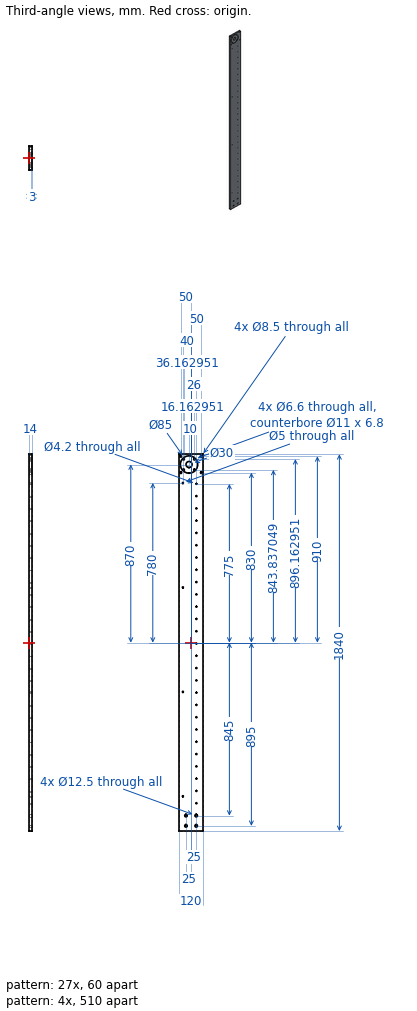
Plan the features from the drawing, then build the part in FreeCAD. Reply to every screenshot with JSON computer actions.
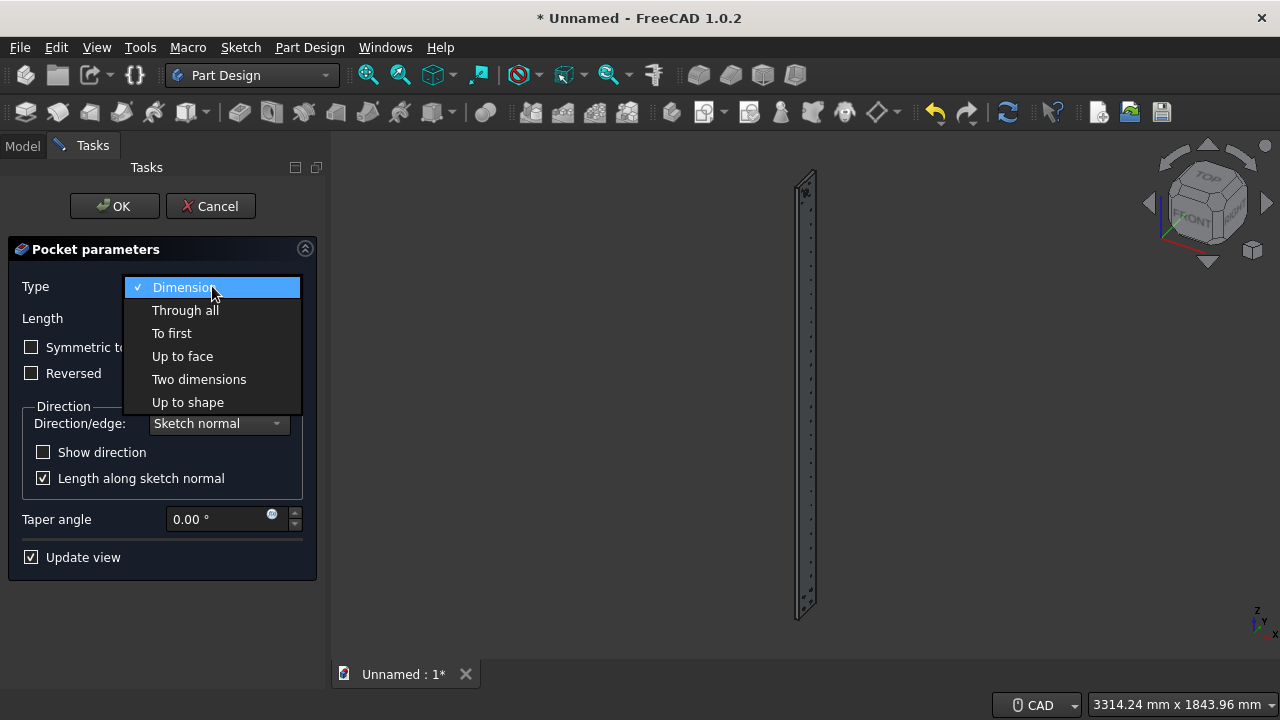
{"action": "left_click", "coordinate": [212, 310]}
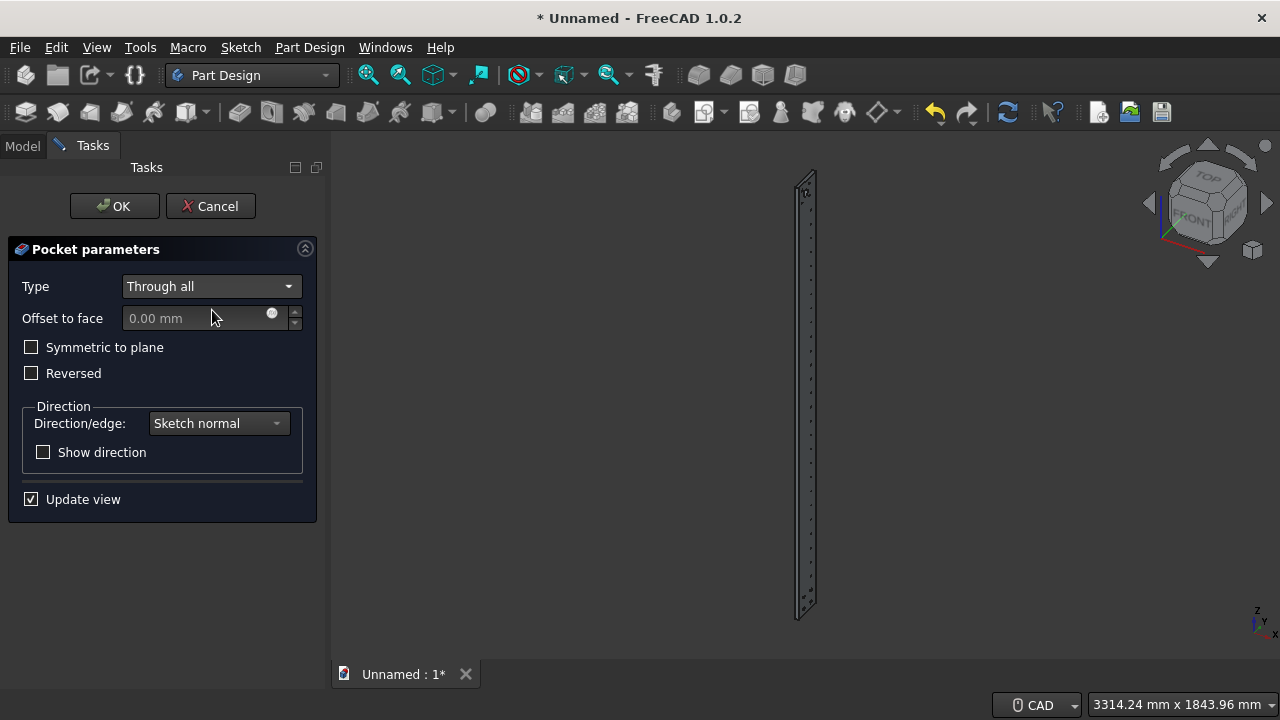
{"action": "left_click", "coordinate": [115, 206]}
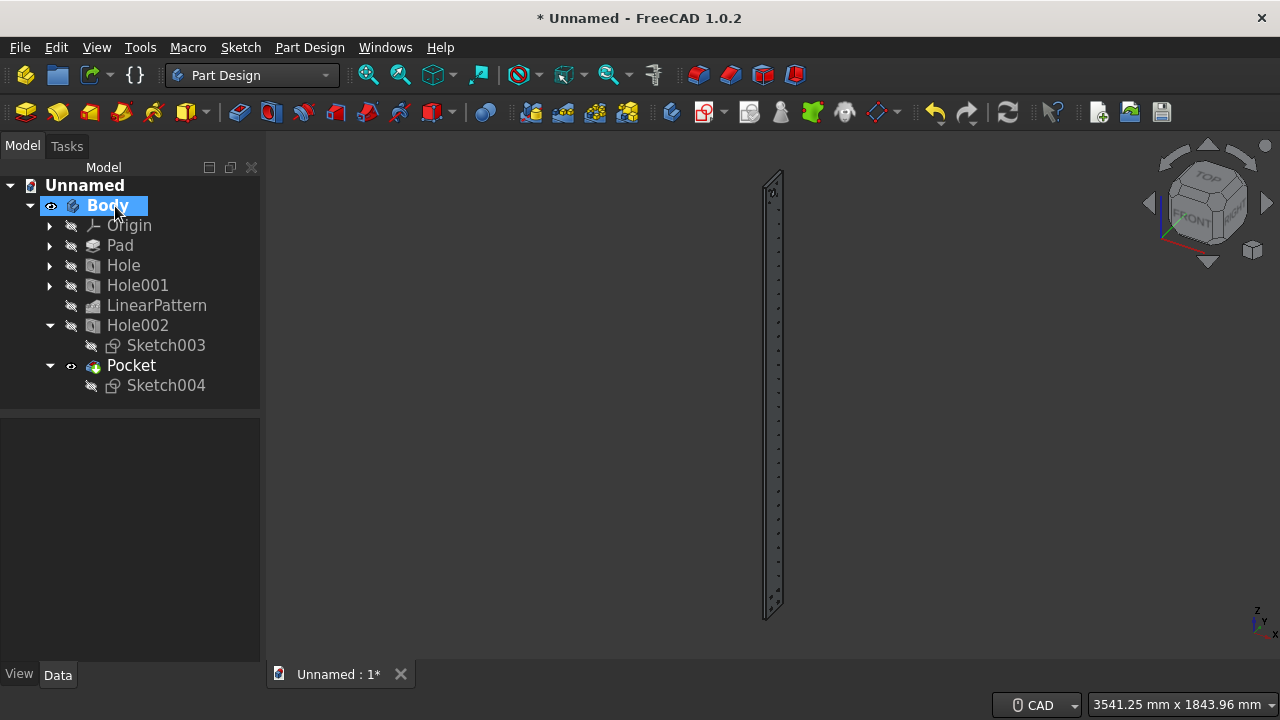
{"action": "key", "text": "6"}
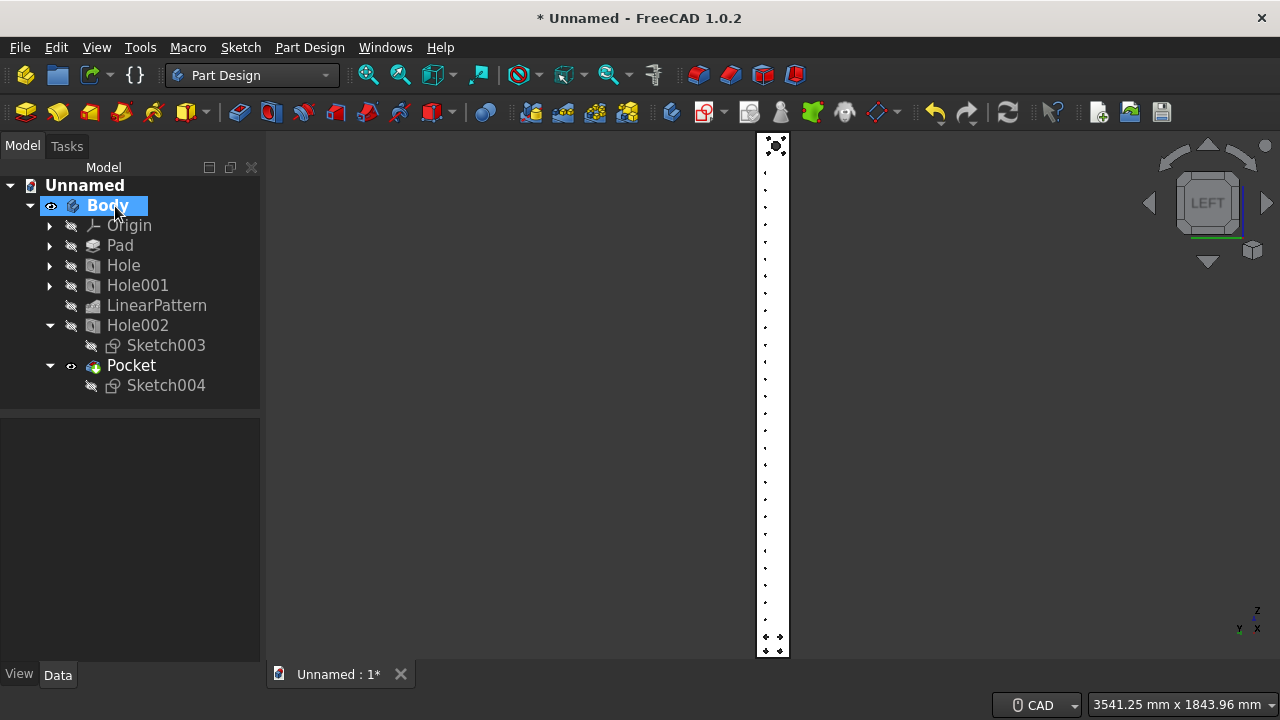
{"action": "left_click", "coordinate": [778, 545]}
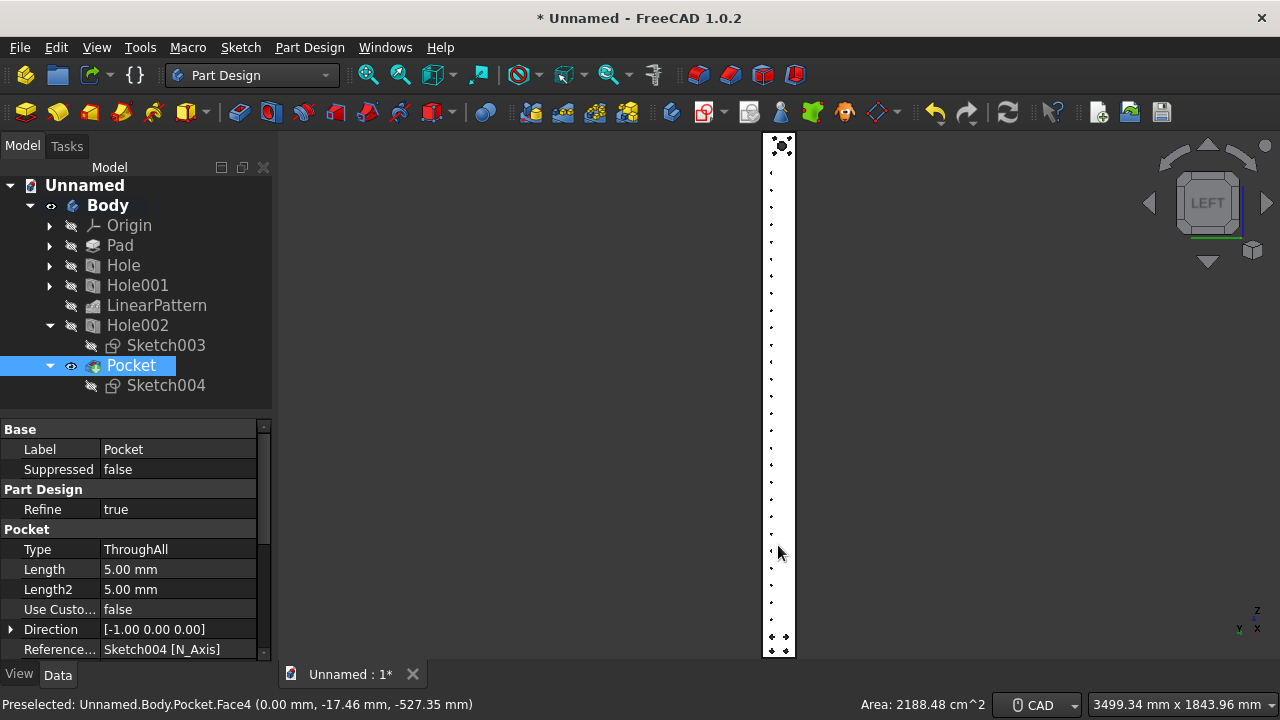
{"action": "left_click", "coordinate": [704, 112]}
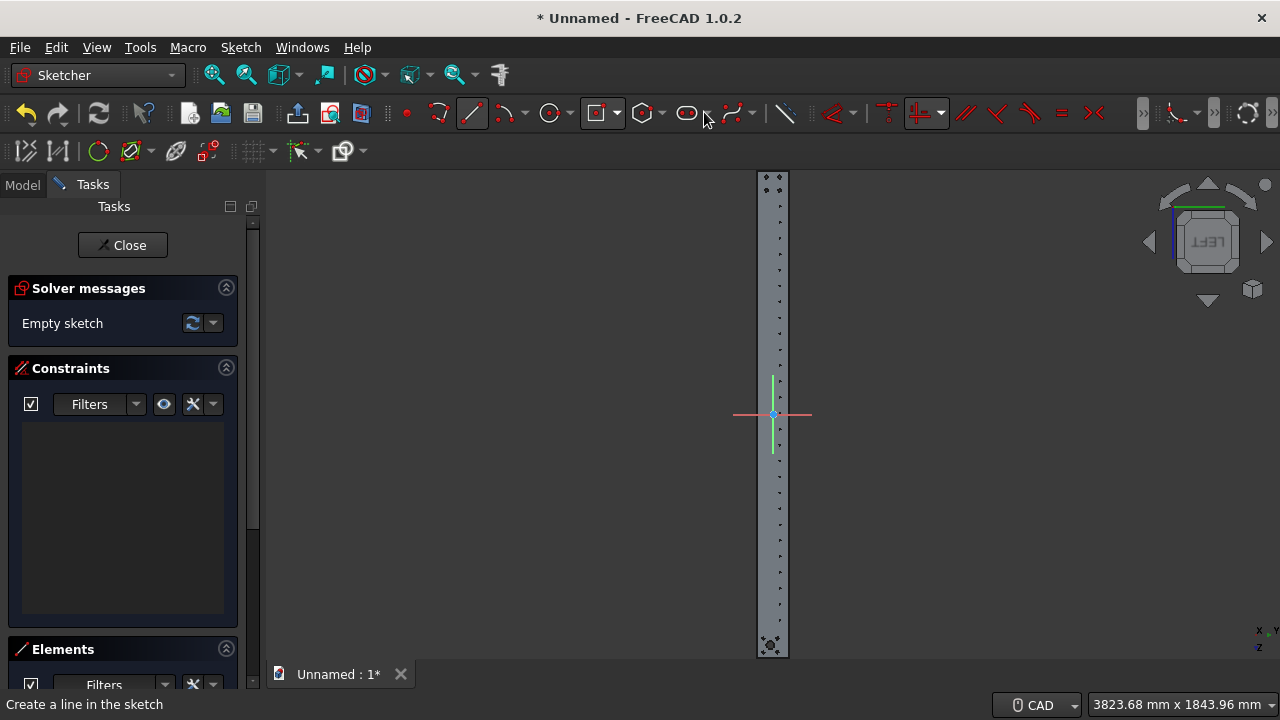
{"action": "scroll", "coordinate": [765, 631], "scroll_direction": "up", "scroll_amount": 15}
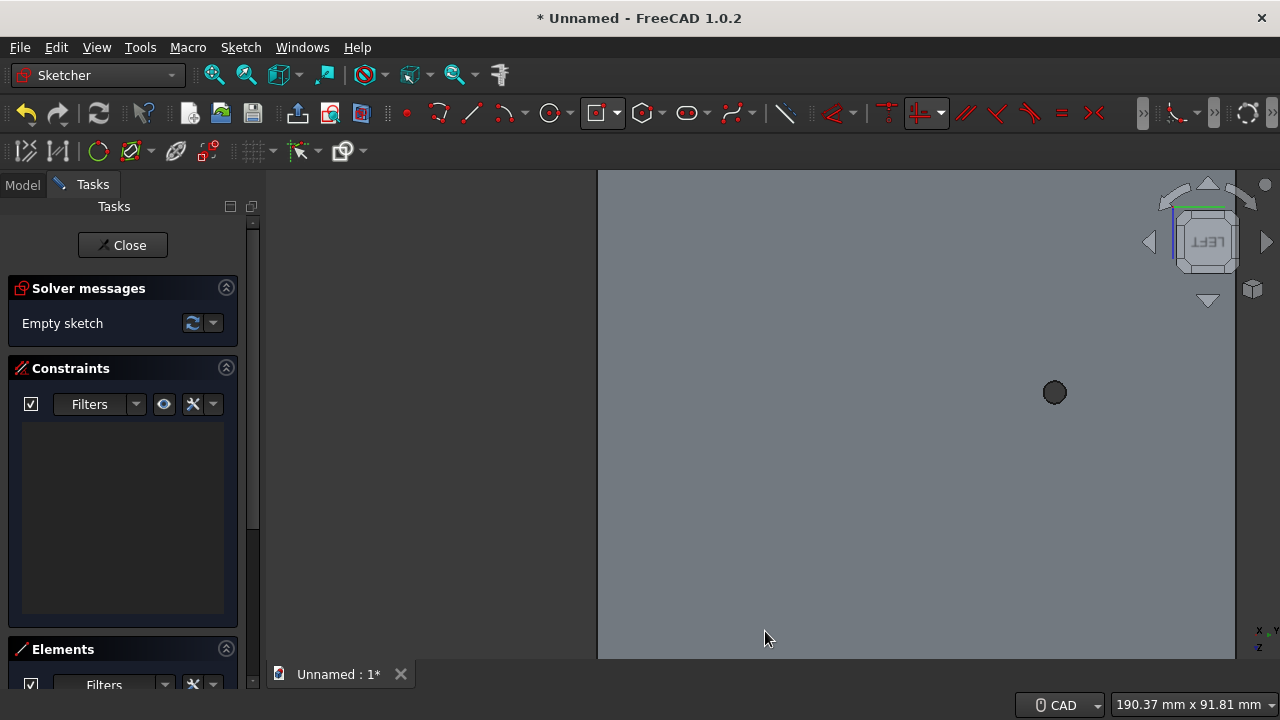
{"action": "scroll", "coordinate": [703, 420], "scroll_direction": "up", "scroll_amount": 12}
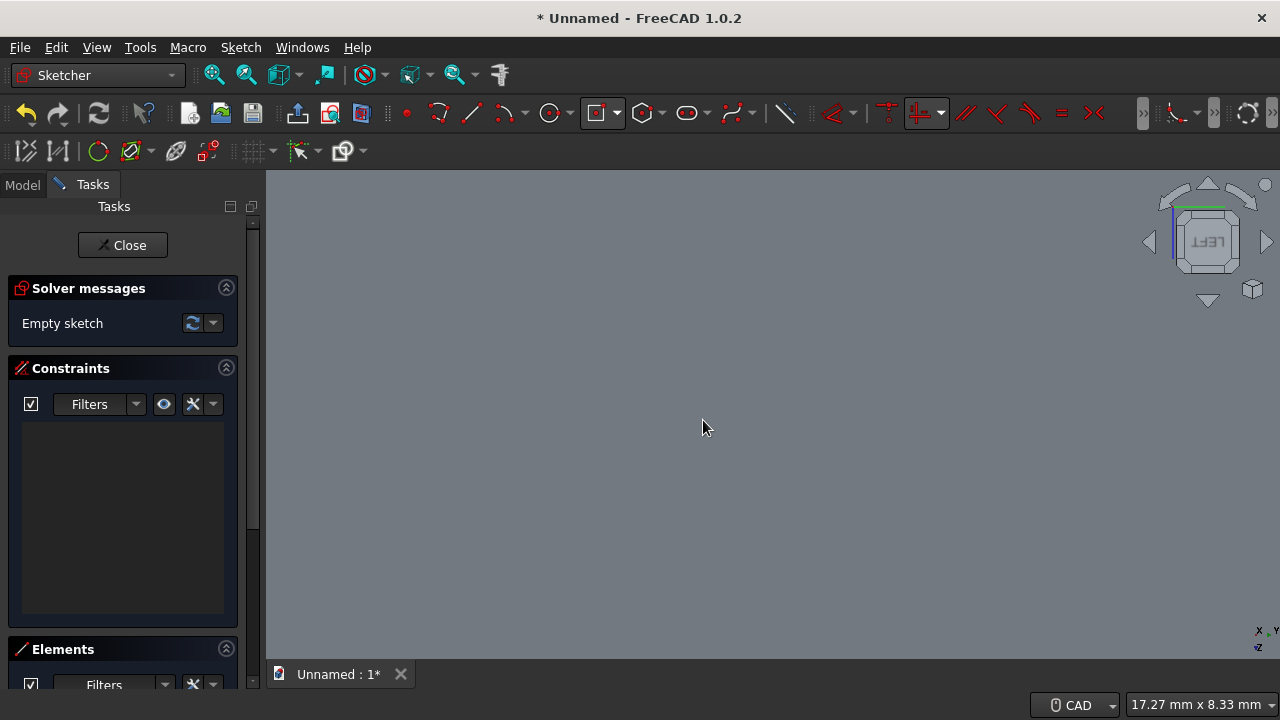
{"action": "left_click", "coordinate": [550, 114]}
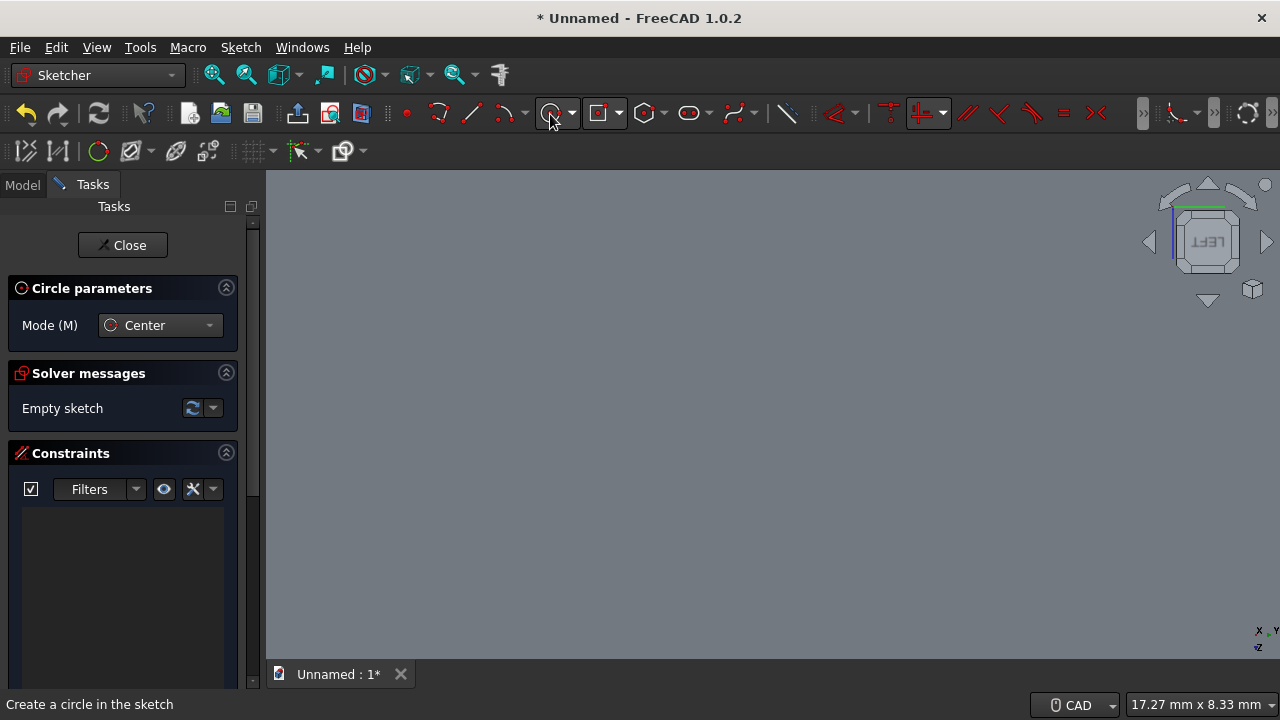
{"action": "left_click", "coordinate": [701, 405]}
{"action": "mouse_move", "coordinate": [805, 301]}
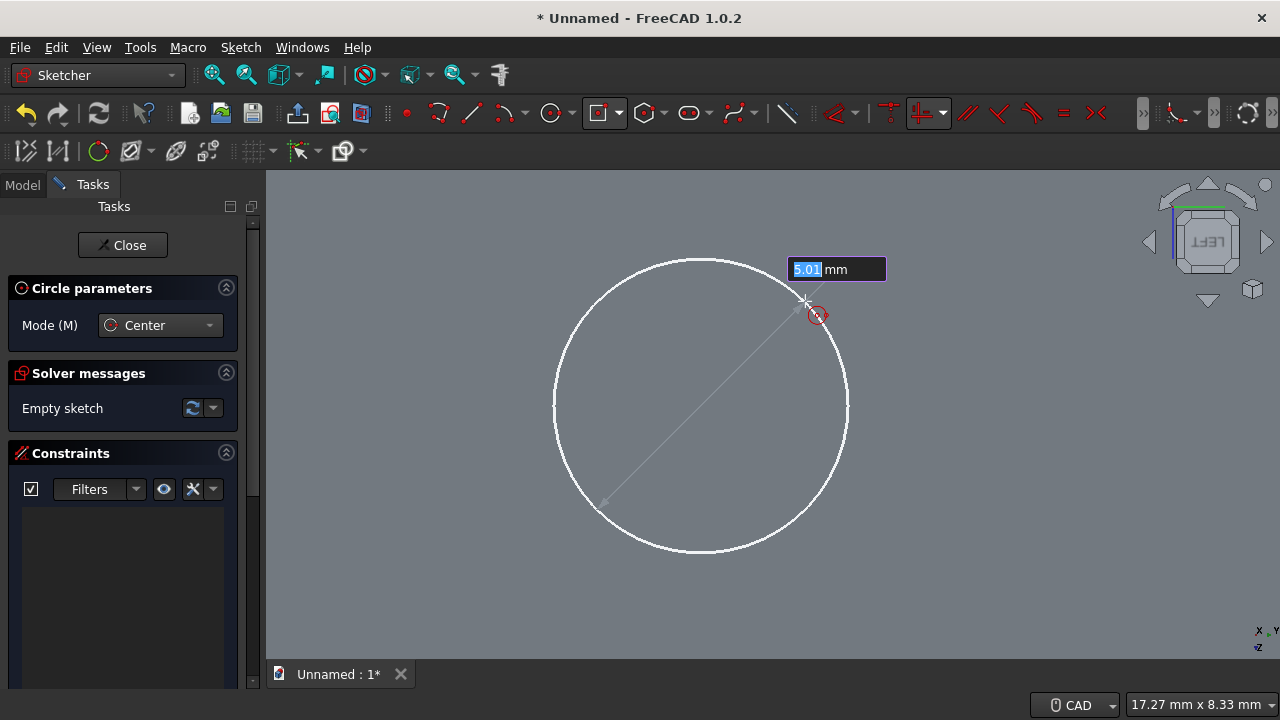
{"action": "type", "text": "5"}
{"action": "key", "text": "Return"}
{"action": "key", "text": "Escape"}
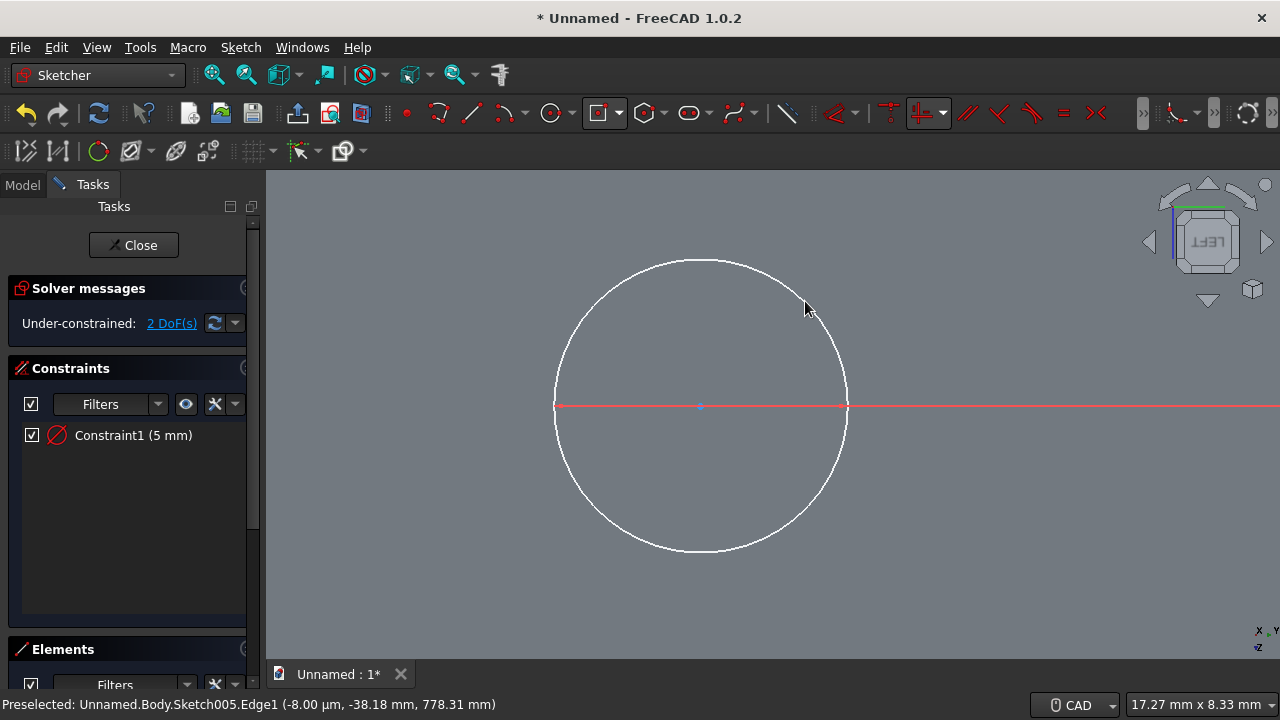
{"action": "left_click", "coordinate": [834, 114]}